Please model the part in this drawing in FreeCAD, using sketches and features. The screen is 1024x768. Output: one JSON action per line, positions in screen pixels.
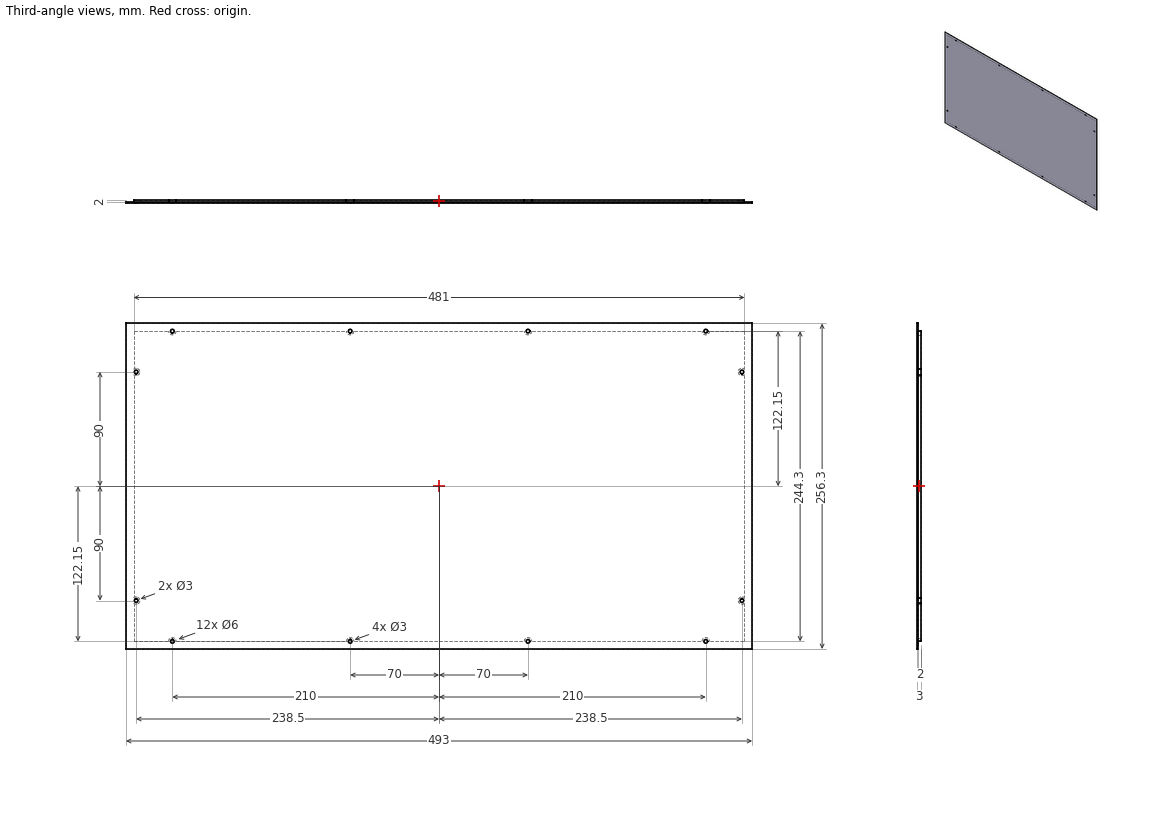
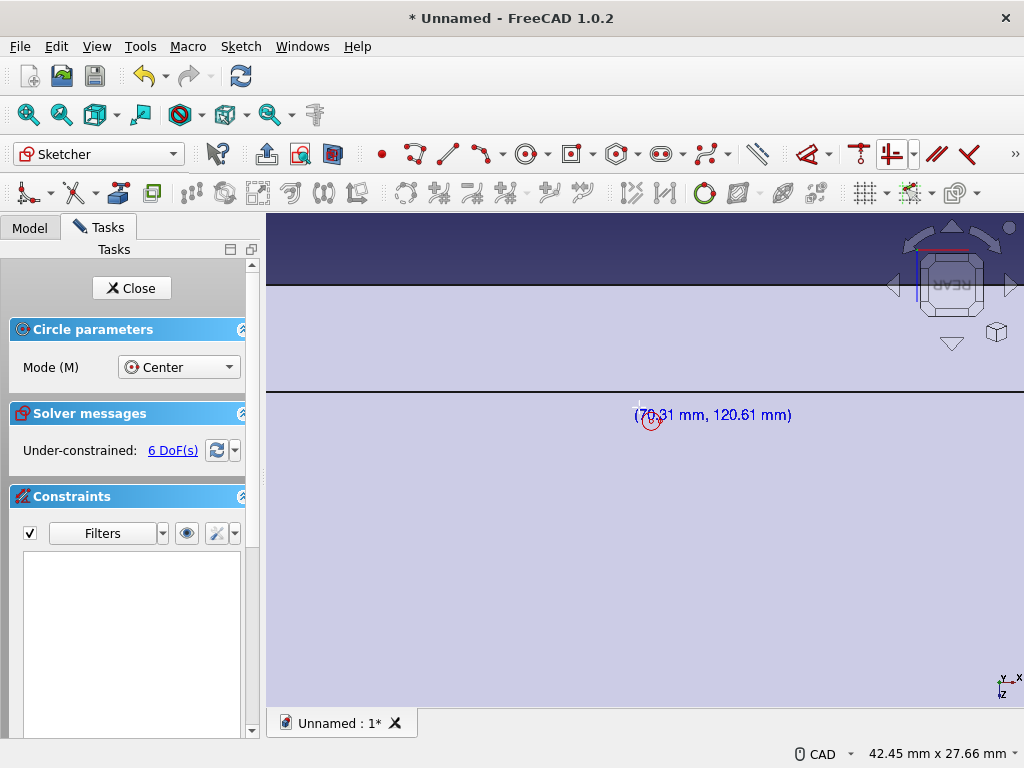
{"action": "scroll", "coordinate": [639, 407], "scroll_direction": "down", "scroll_amount": 15}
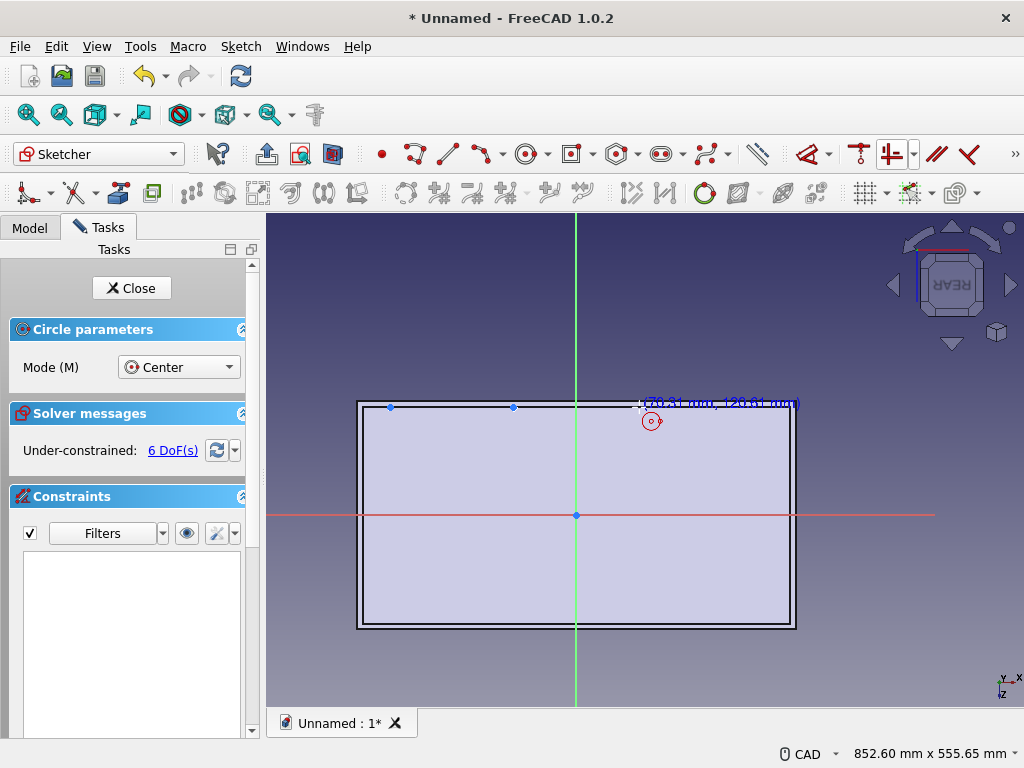
{"action": "left_click", "coordinate": [639, 407]}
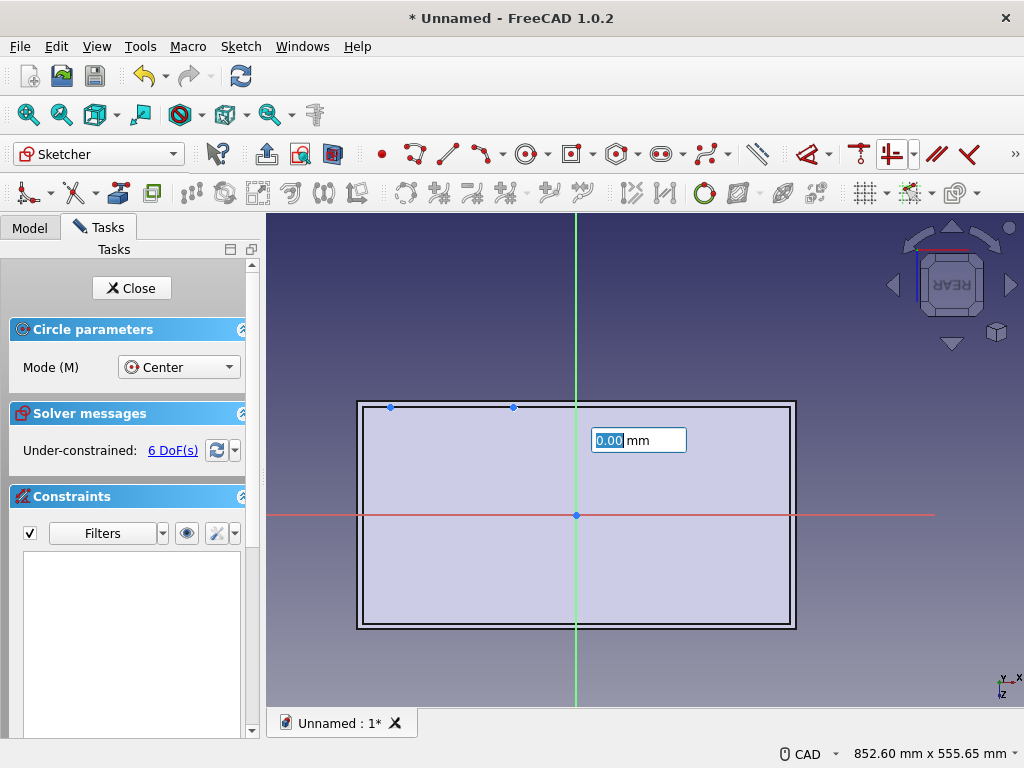
{"action": "scroll", "coordinate": [640, 406], "scroll_direction": "up", "scroll_amount": 13}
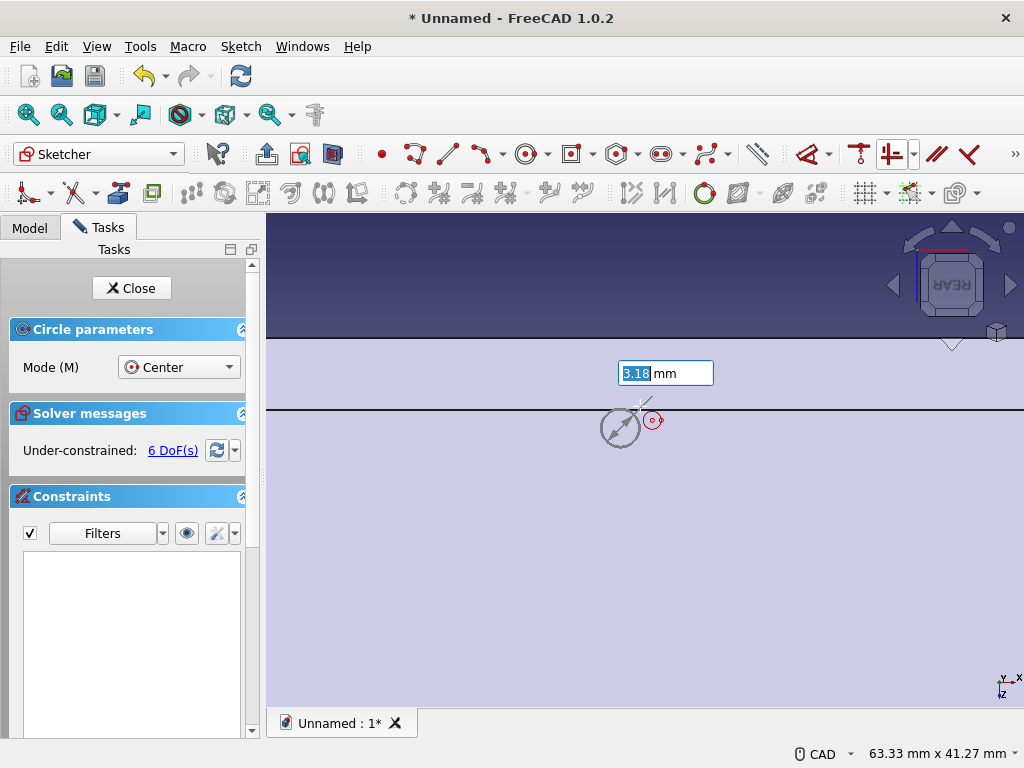
{"action": "left_click", "coordinate": [629, 397]}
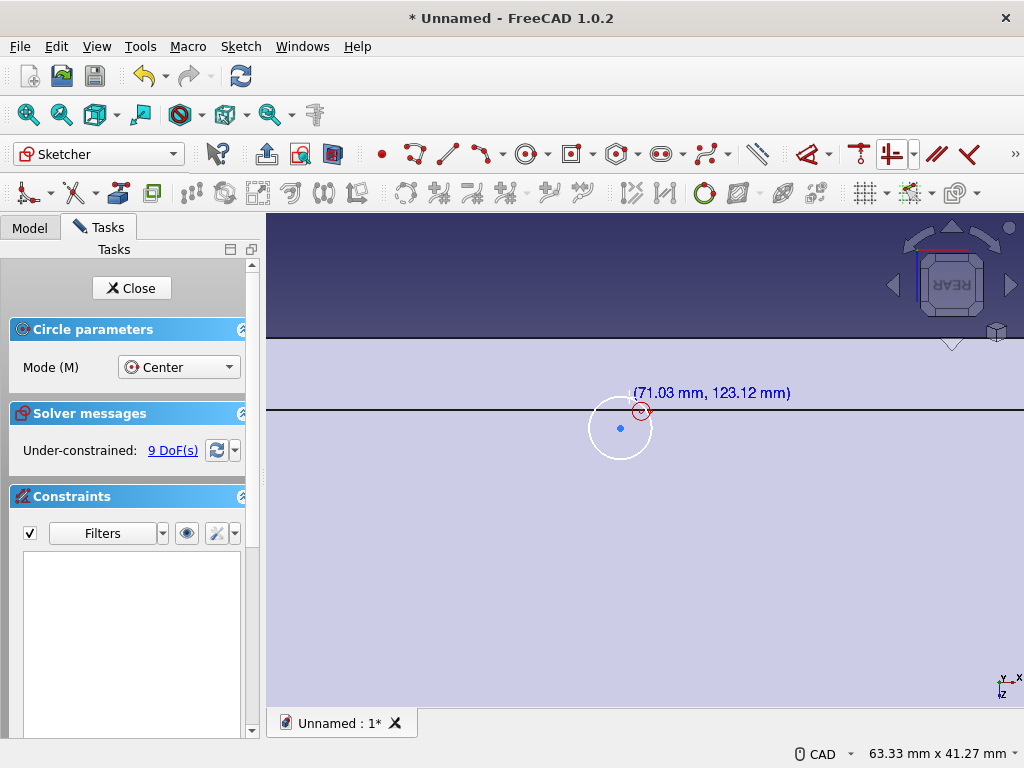
{"action": "scroll", "coordinate": [641, 406], "scroll_direction": "down", "scroll_amount": 13}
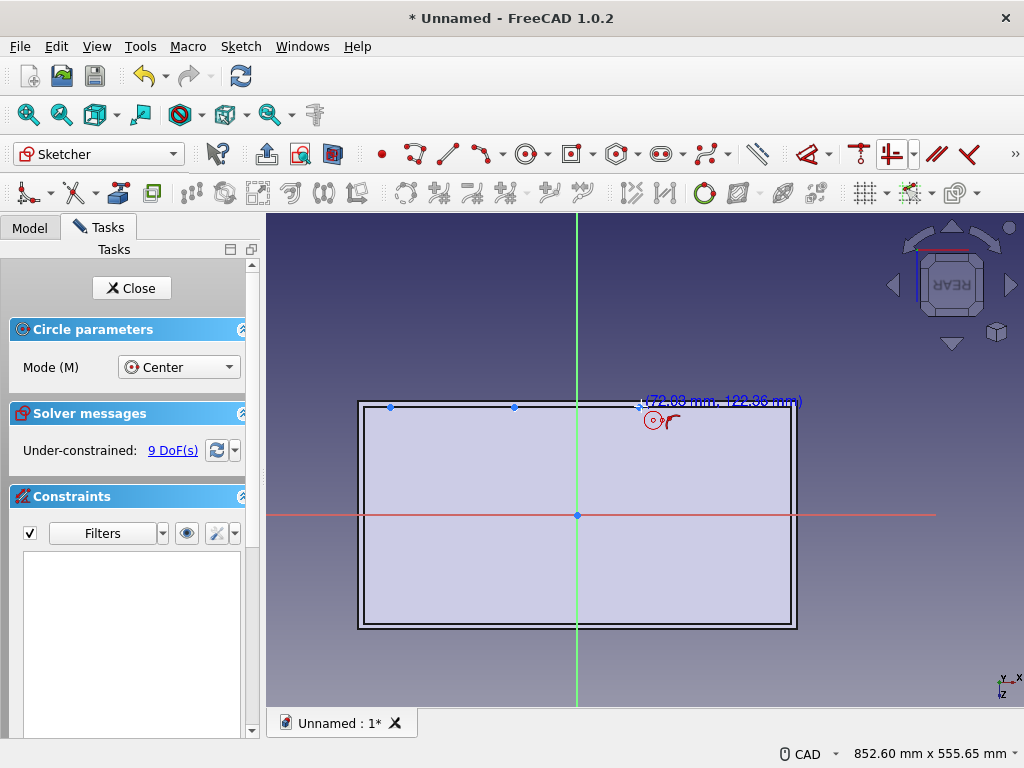
{"action": "scroll", "coordinate": [764, 407], "scroll_direction": "up", "scroll_amount": 15}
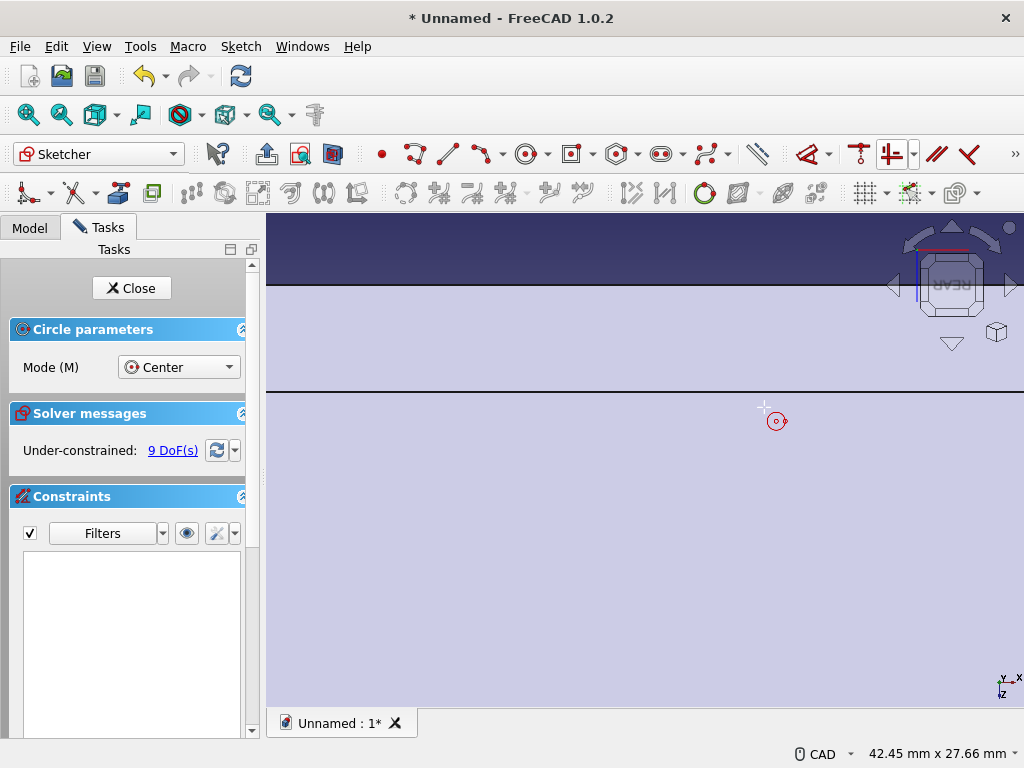
{"action": "scroll", "coordinate": [764, 407], "scroll_direction": "down", "scroll_amount": 15}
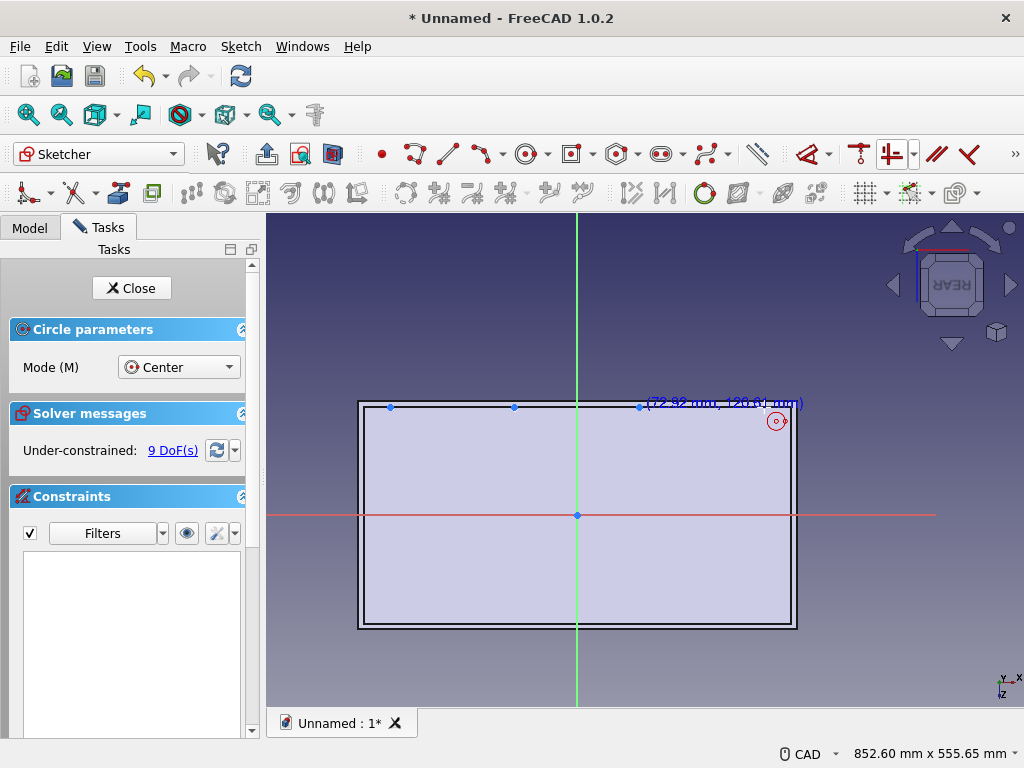
{"action": "left_click", "coordinate": [764, 407]}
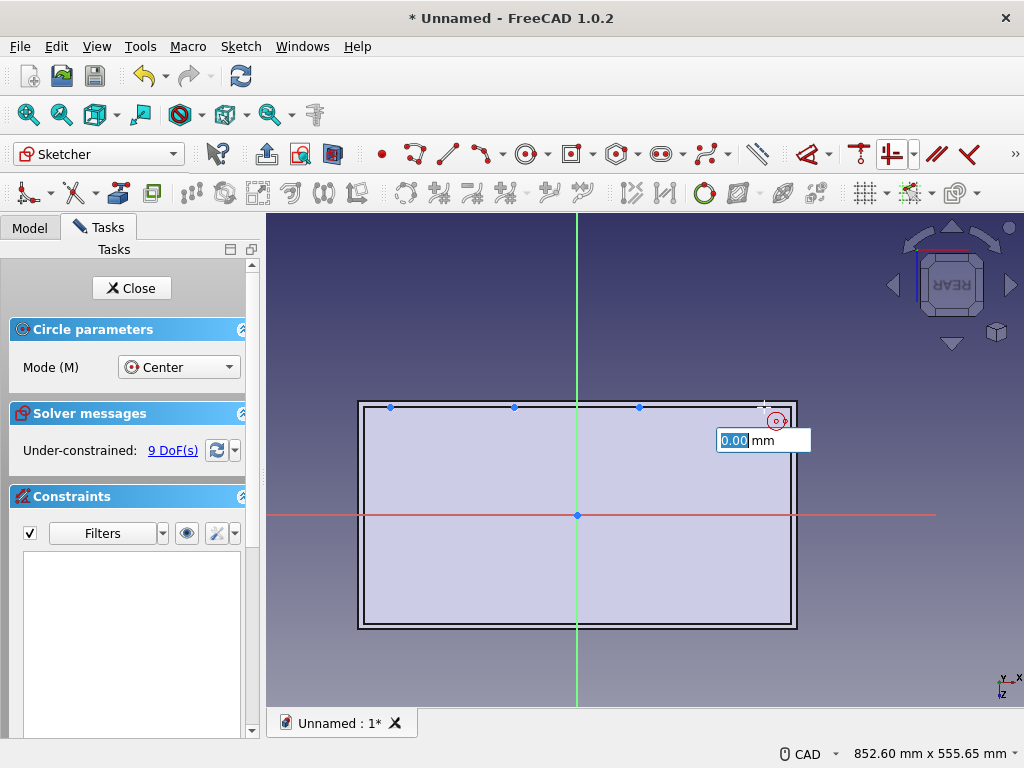
{"action": "scroll", "coordinate": [765, 406], "scroll_direction": "up", "scroll_amount": 13}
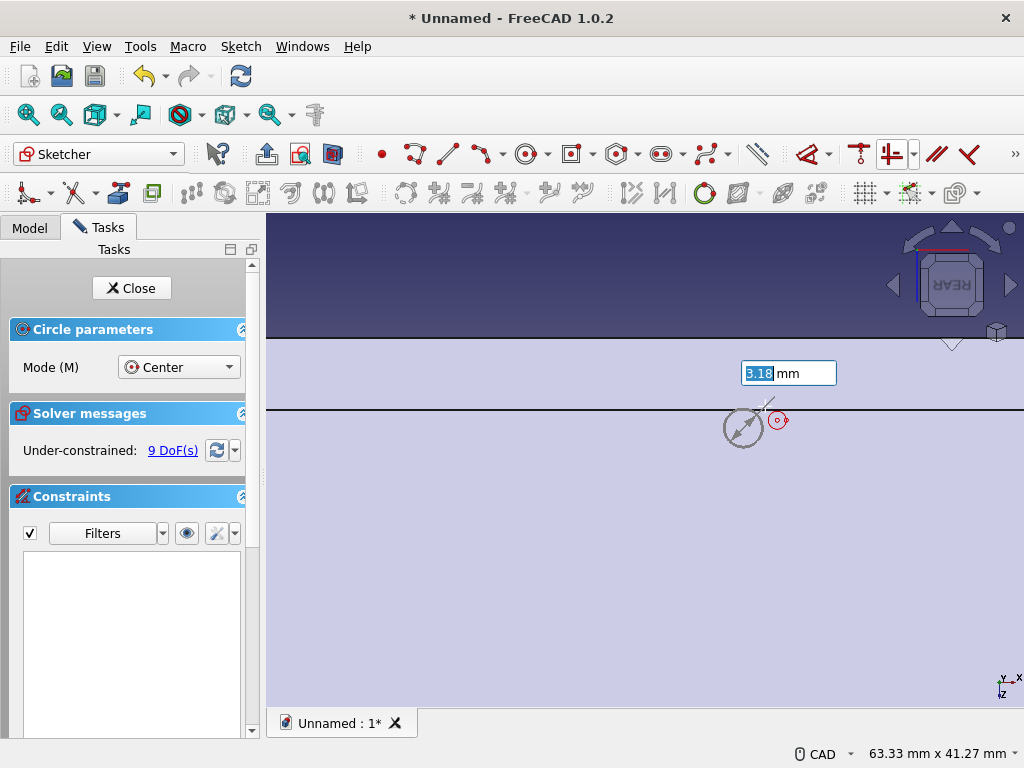
{"action": "left_click", "coordinate": [758, 397]}
{"action": "key", "text": "Escape"}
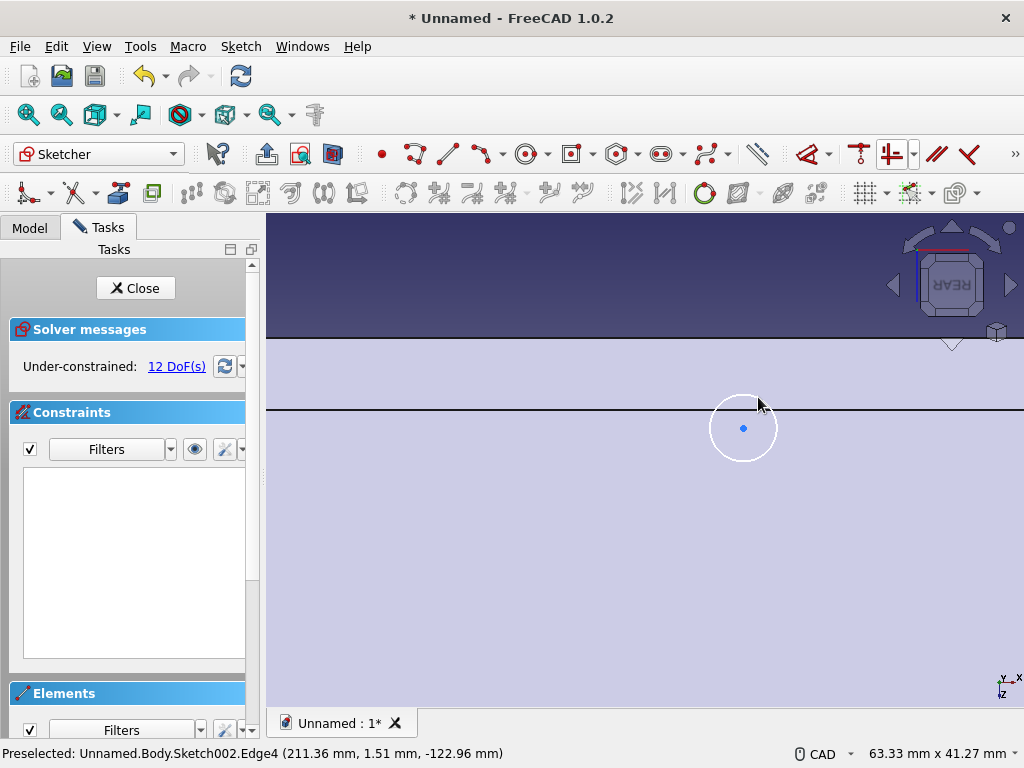
{"action": "scroll", "coordinate": [765, 406], "scroll_direction": "down", "scroll_amount": 13}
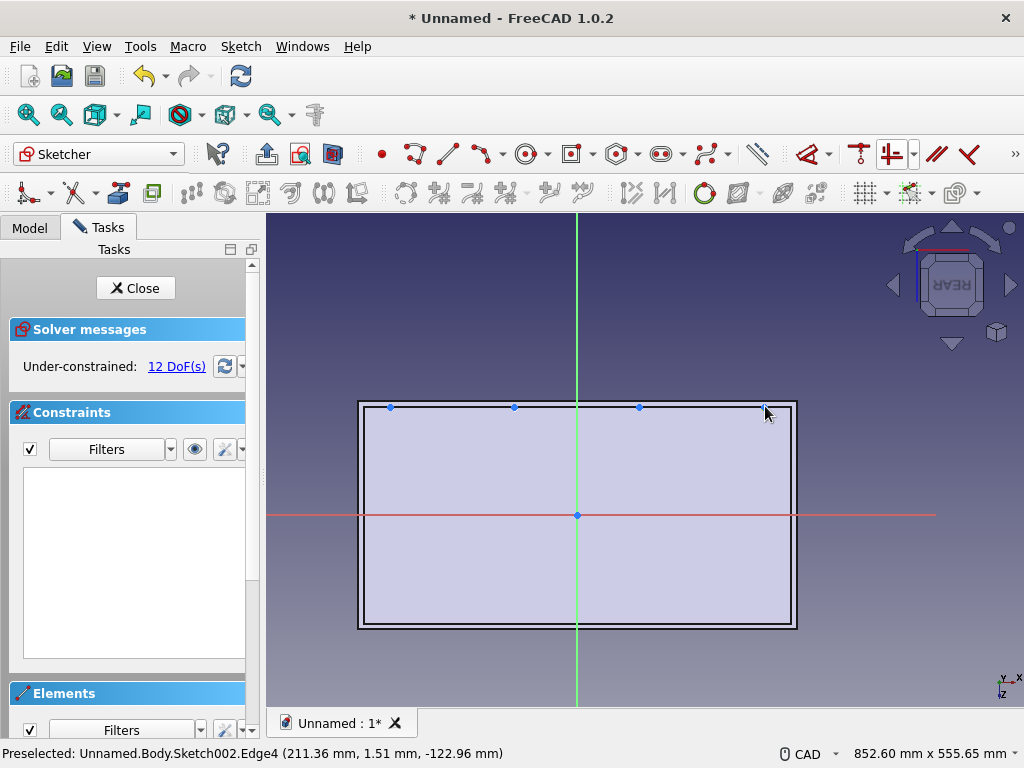
{"action": "scroll", "coordinate": [517, 406], "scroll_direction": "up", "scroll_amount": 9}